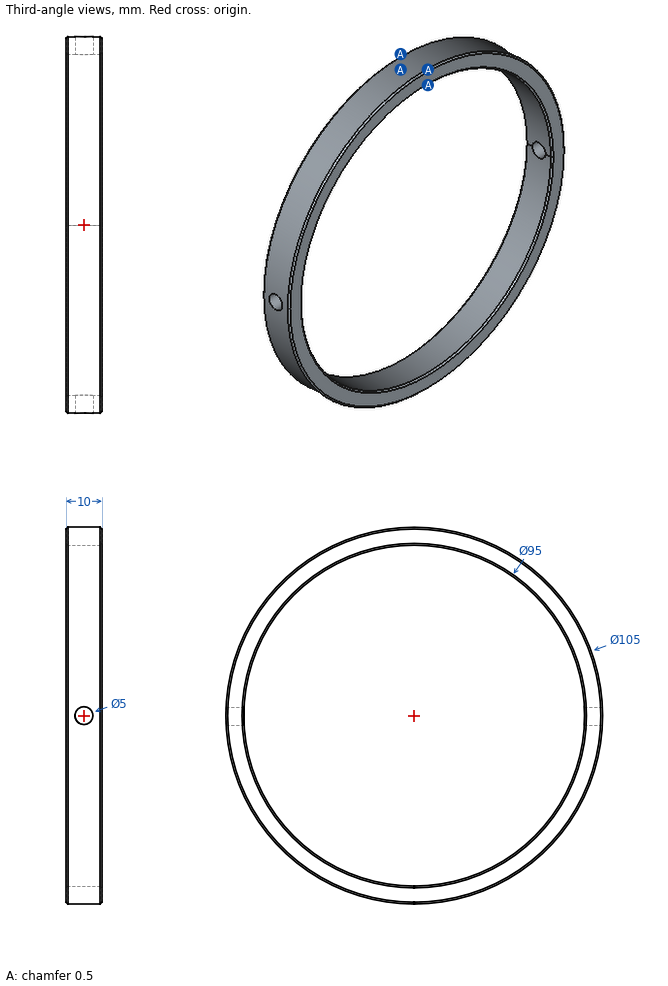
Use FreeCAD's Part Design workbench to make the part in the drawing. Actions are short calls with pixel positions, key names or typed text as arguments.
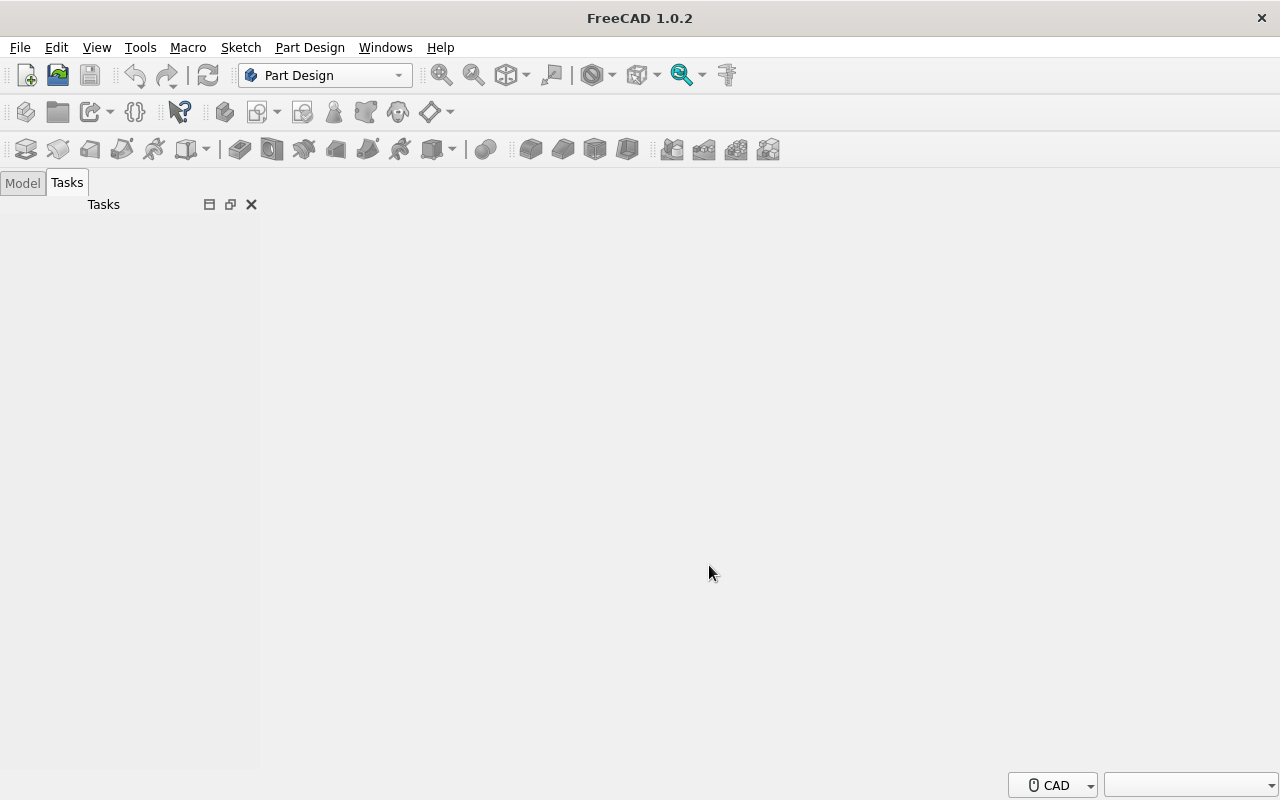
click(26, 76)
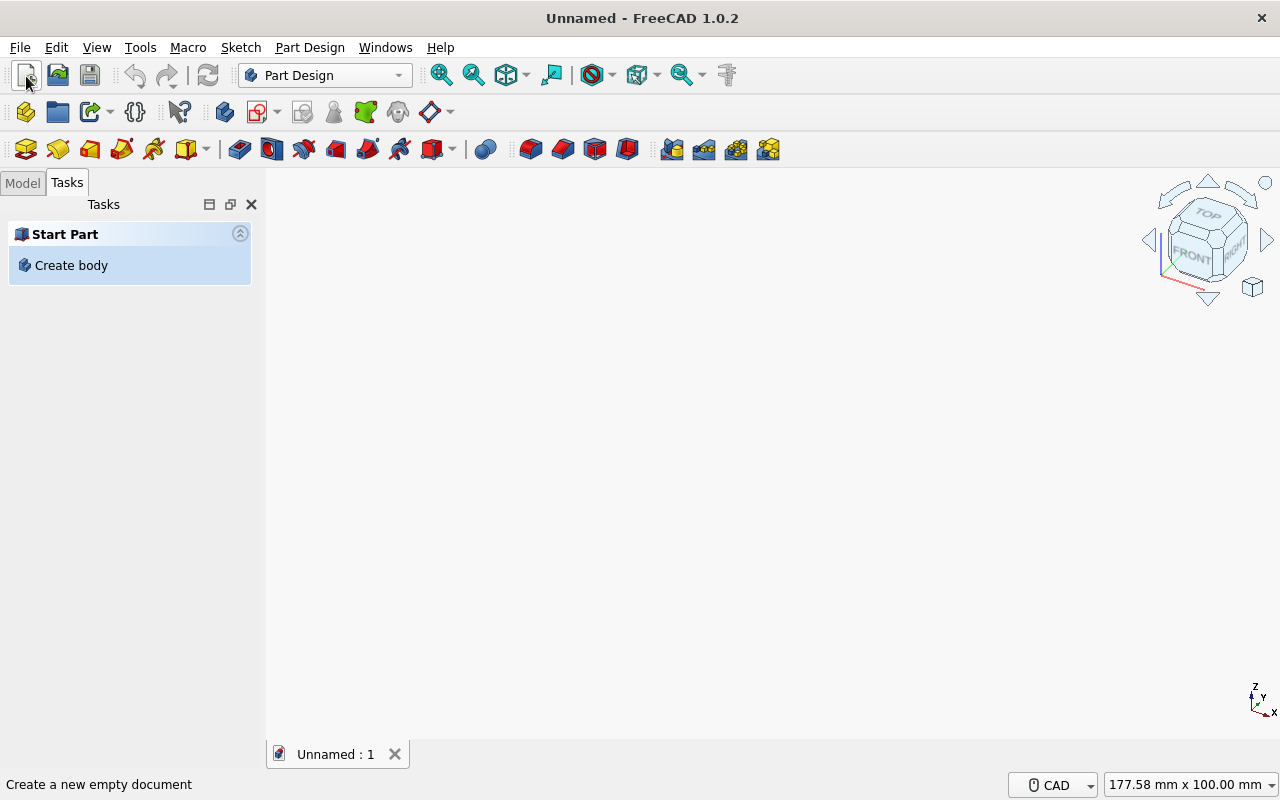
click(258, 112)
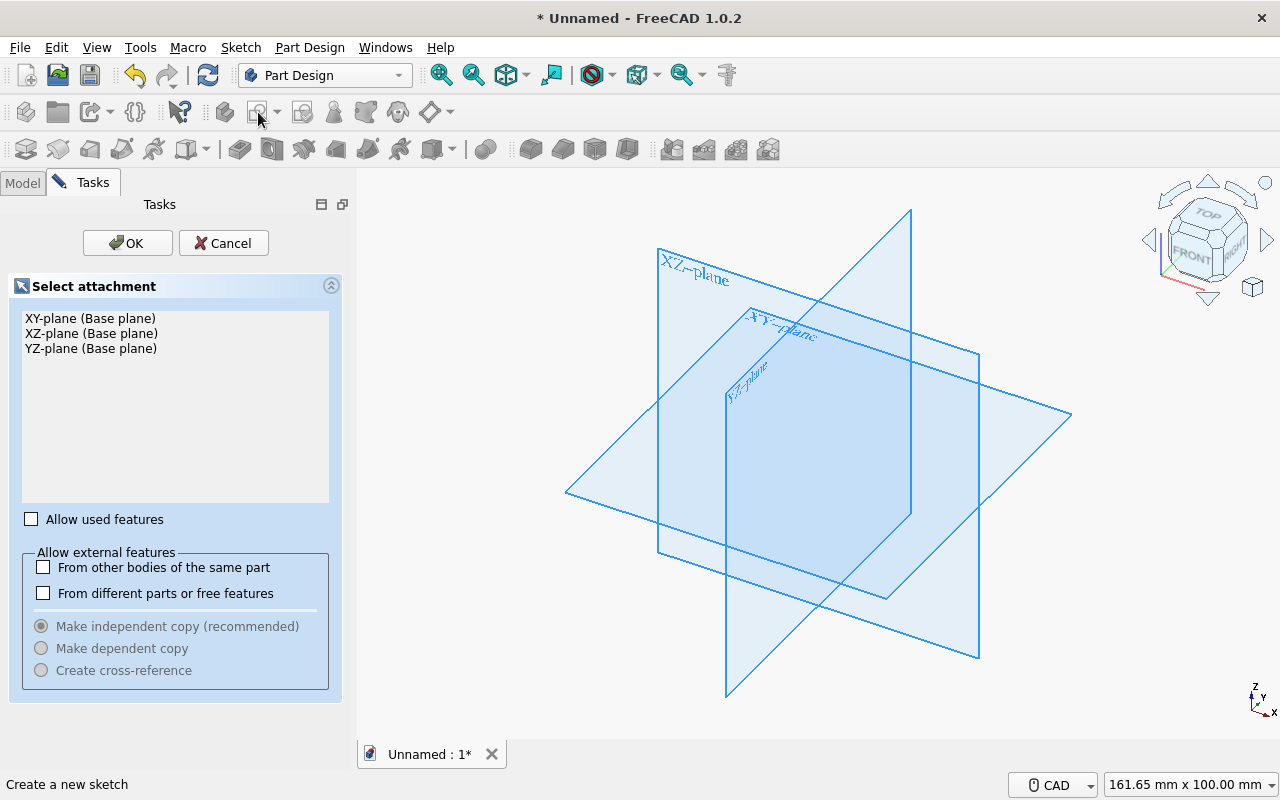
click(82, 348)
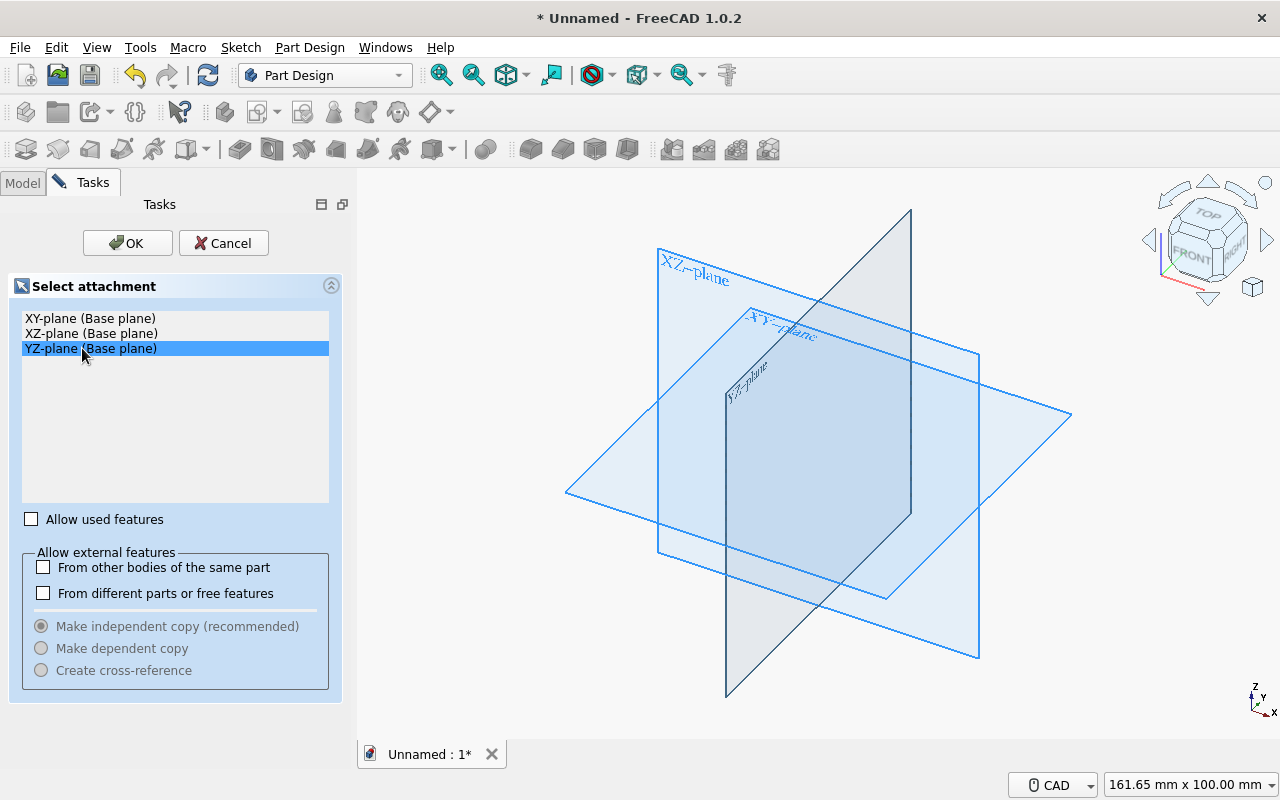
click(128, 243)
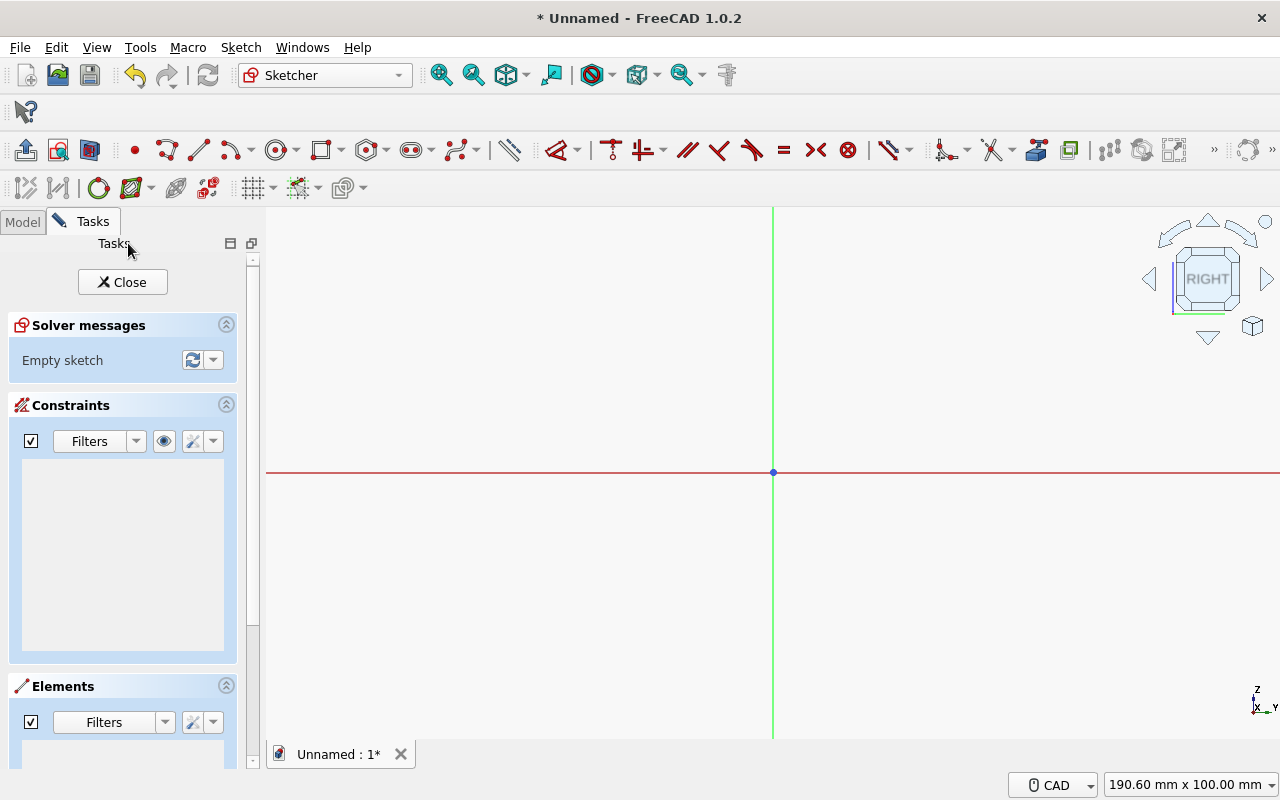
scroll(621, 473, down, 3)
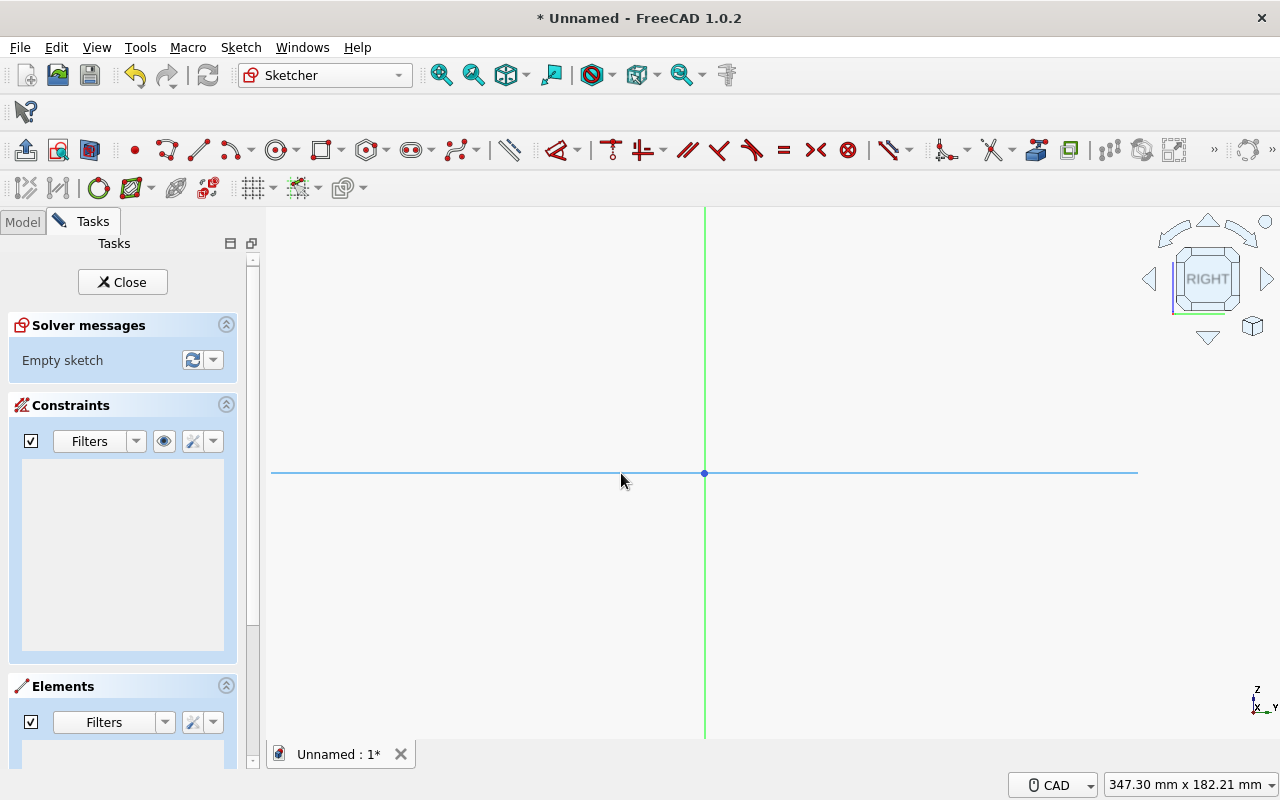
click(276, 150)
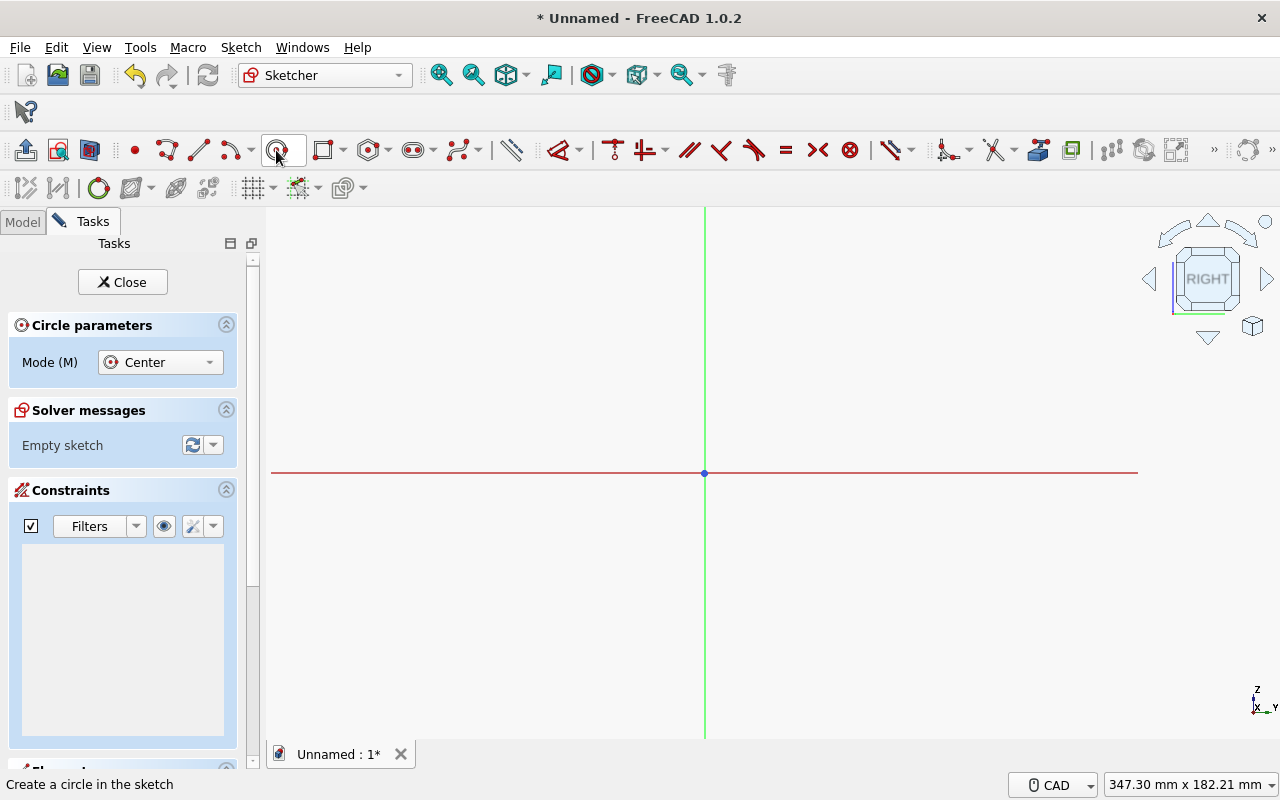
click(705, 473)
click(813, 365)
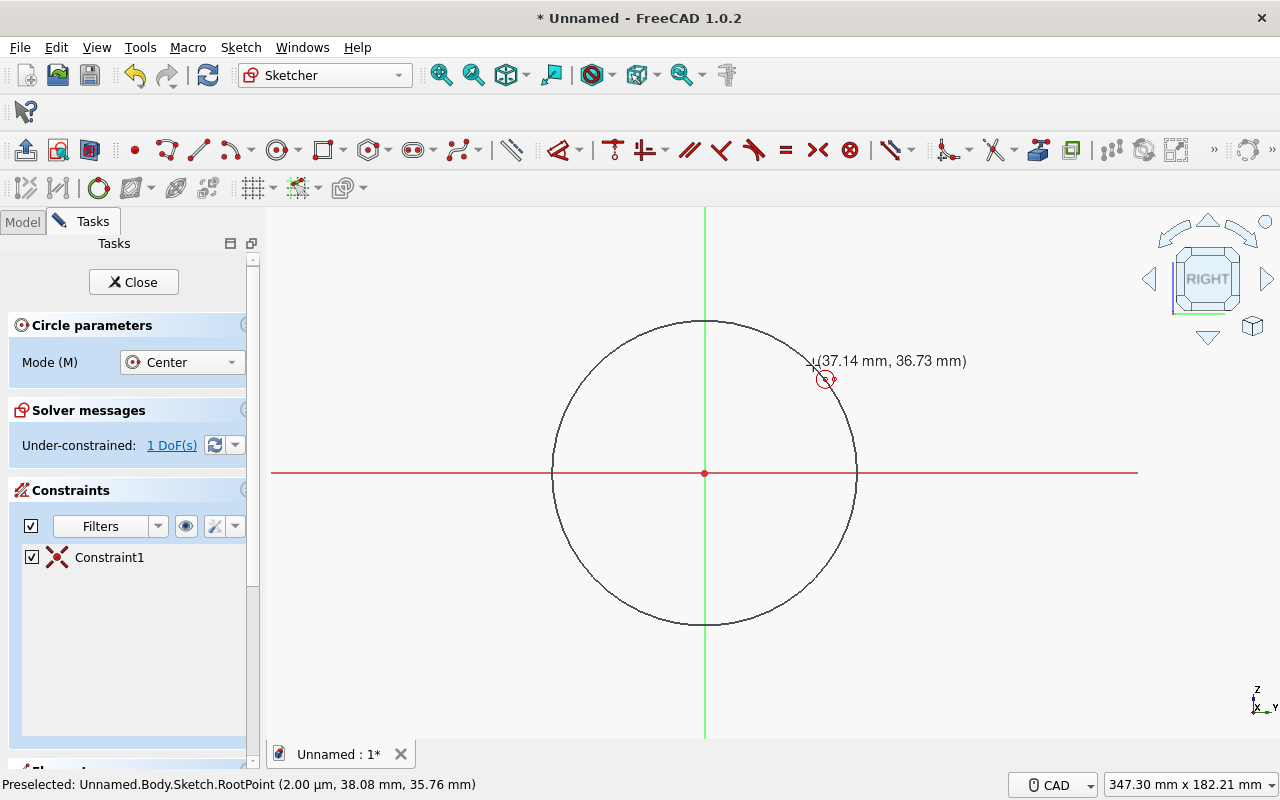
click(705, 473)
click(803, 375)
key(Escape)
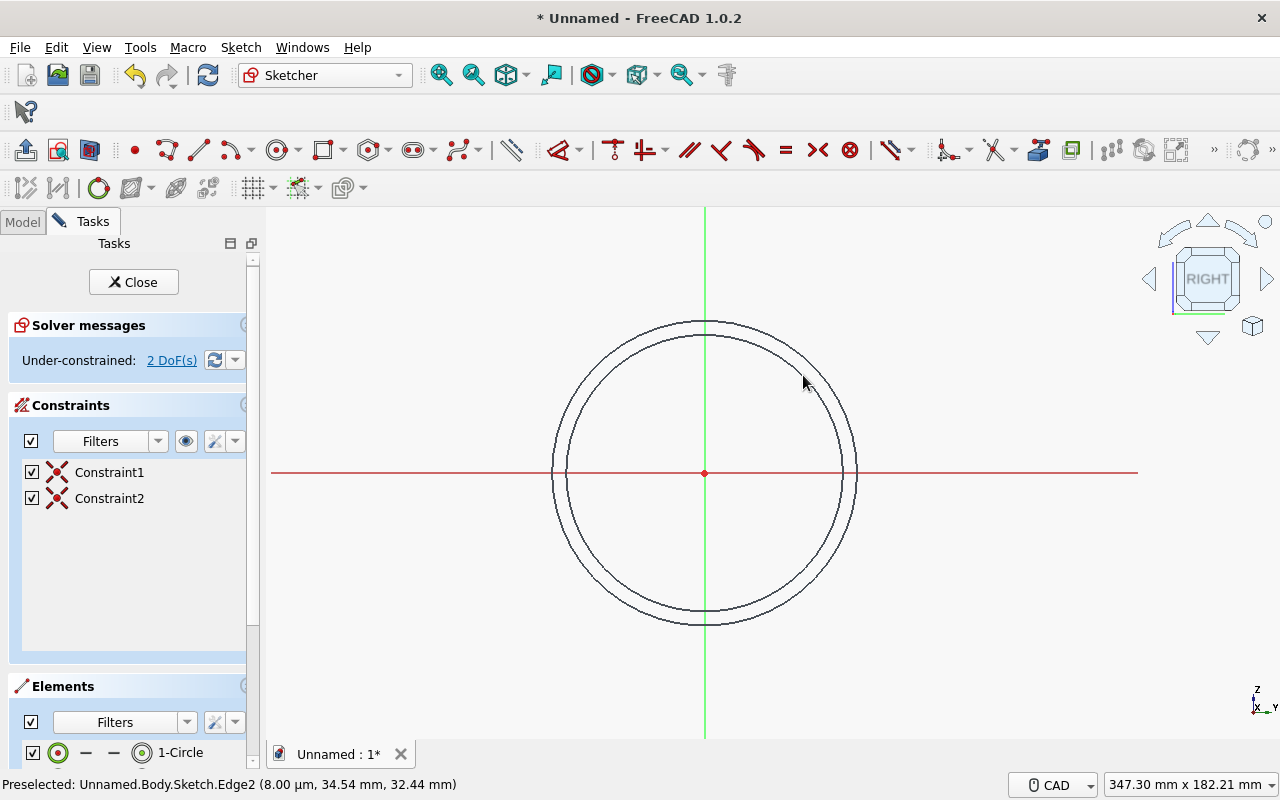
click(558, 150)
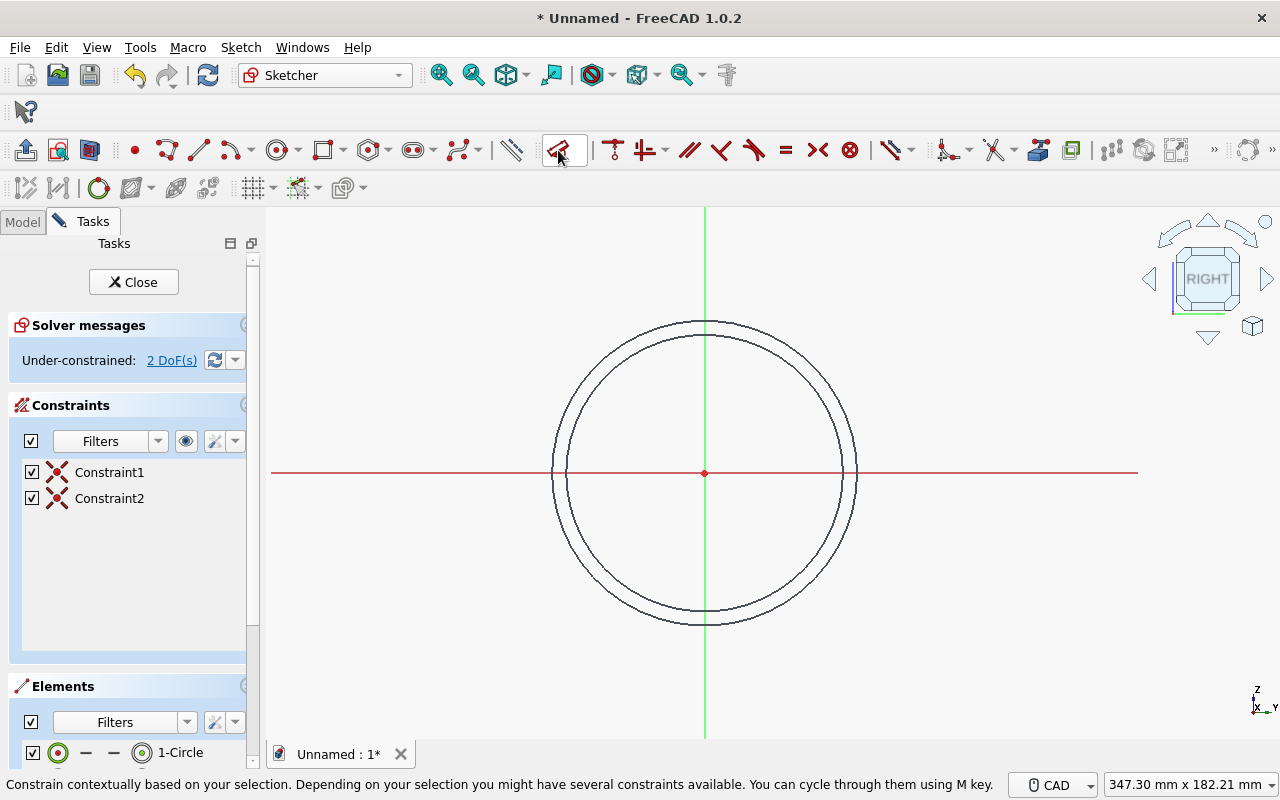
click(812, 365)
click(835, 342)